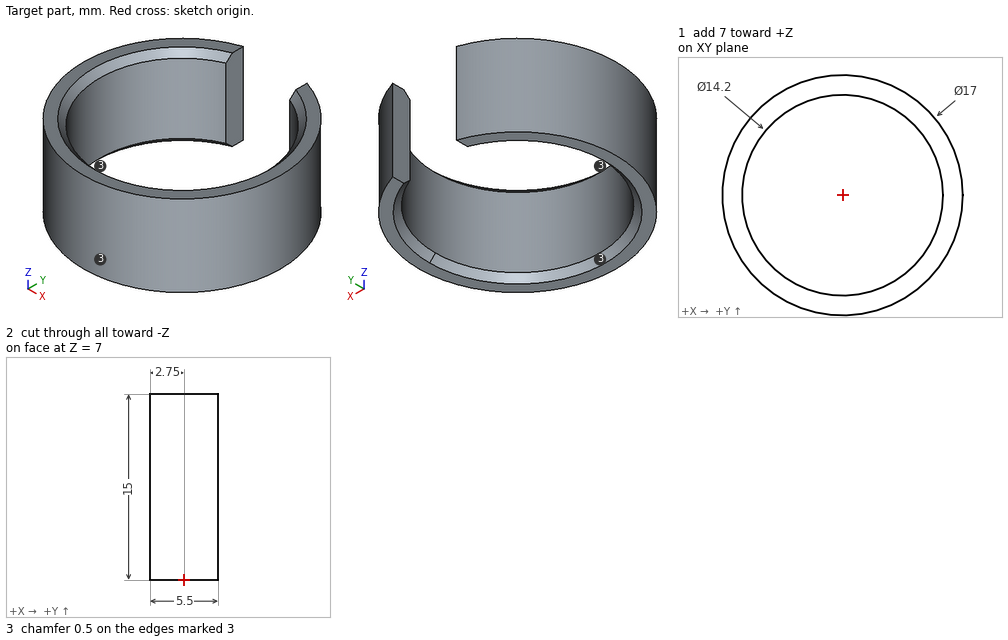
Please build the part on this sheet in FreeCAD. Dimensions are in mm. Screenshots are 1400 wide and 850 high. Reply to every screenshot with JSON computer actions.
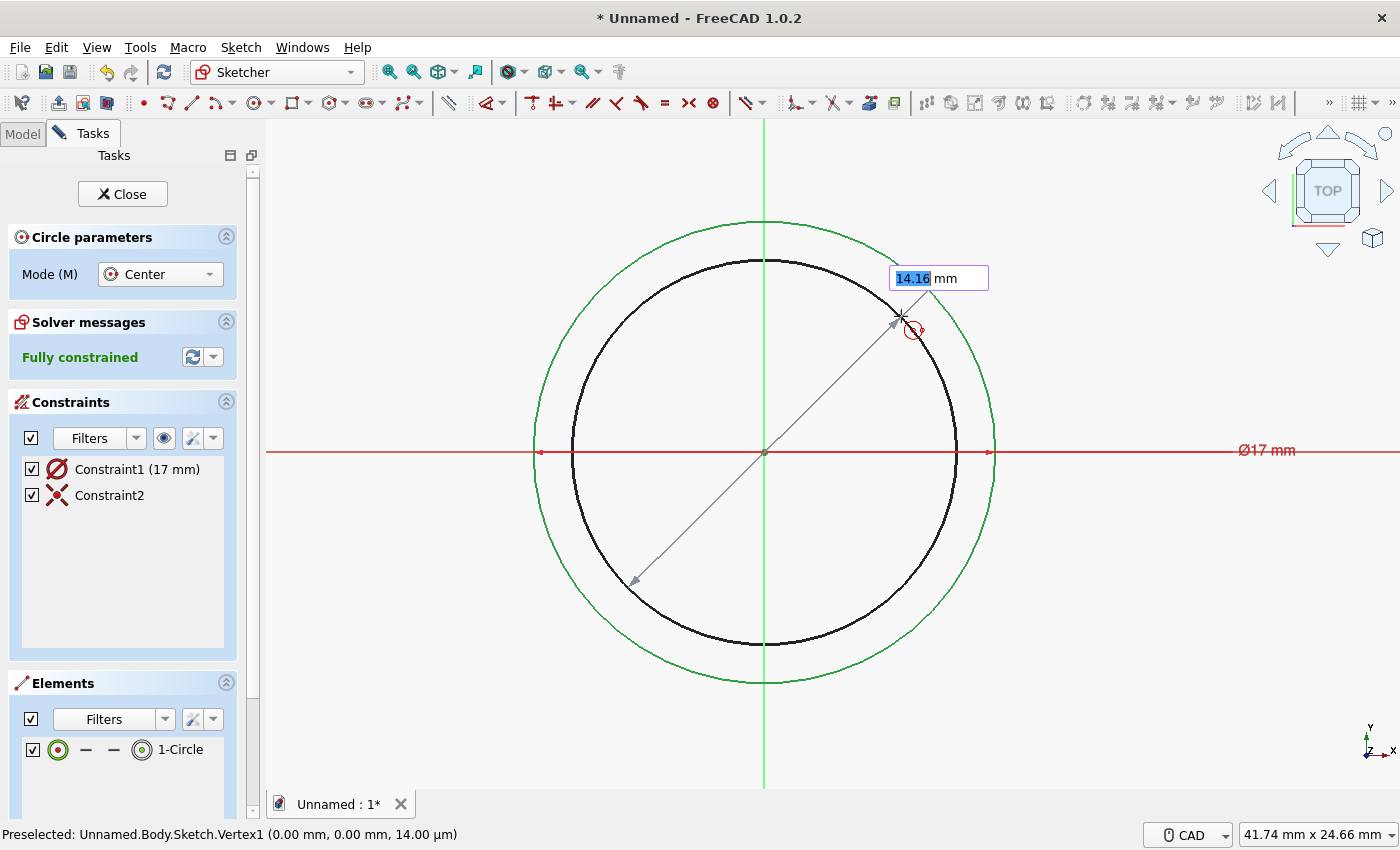
{"action": "type", "text": "14.2"}
{"action": "key", "text": "Return"}
{"action": "key", "text": "Escape"}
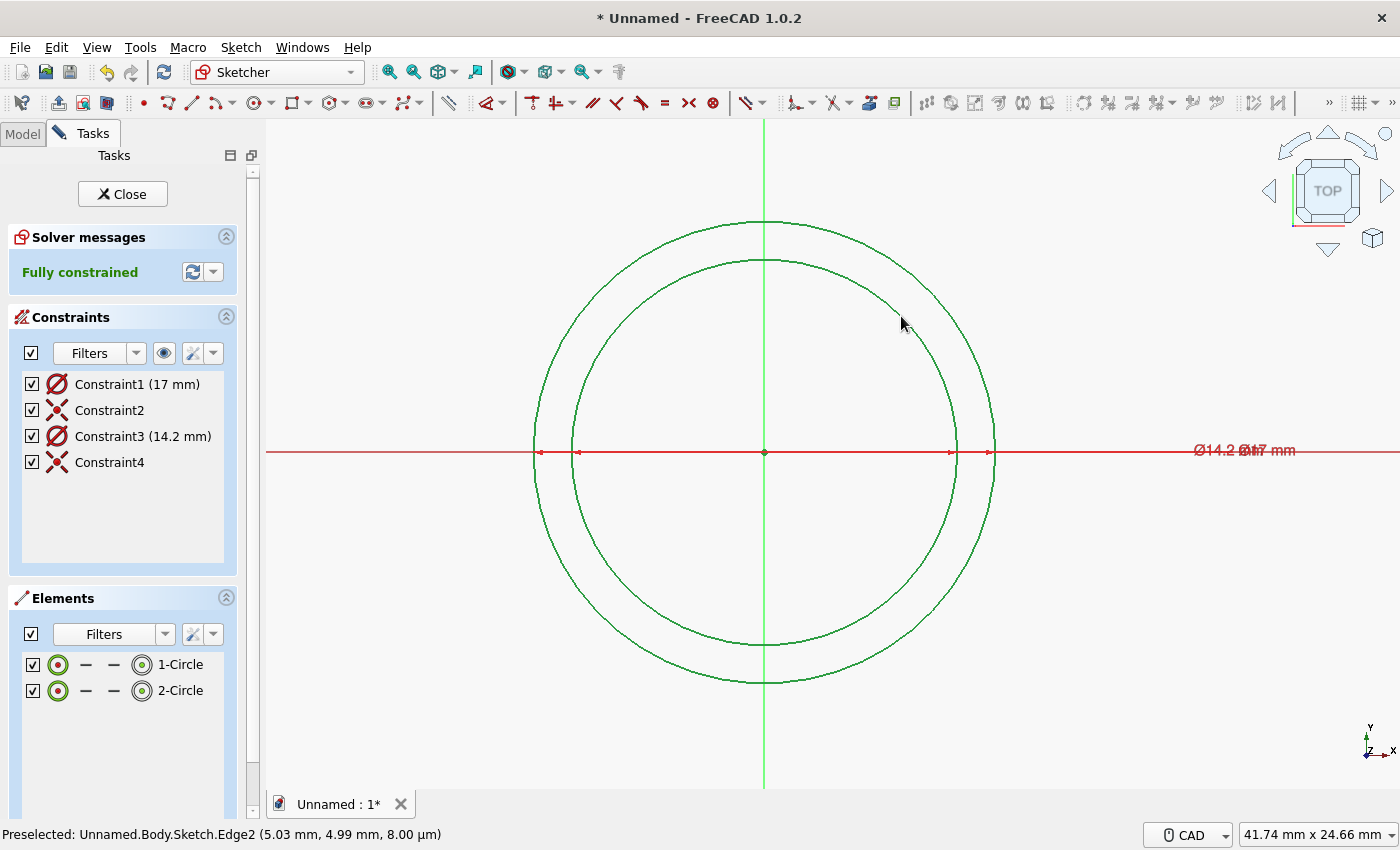
{"action": "left_click", "coordinate": [123, 194]}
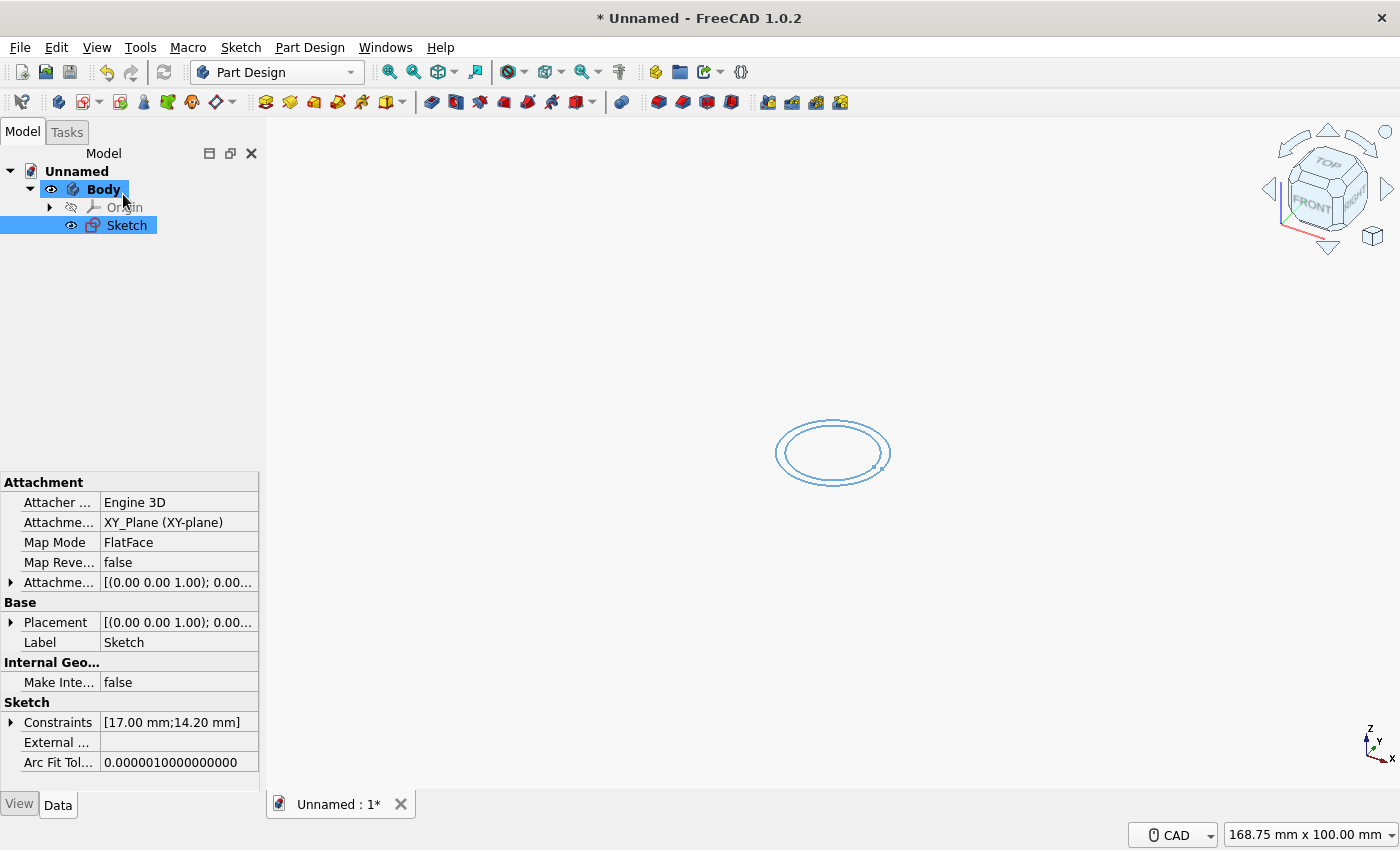
{"action": "left_click", "coordinate": [266, 102]}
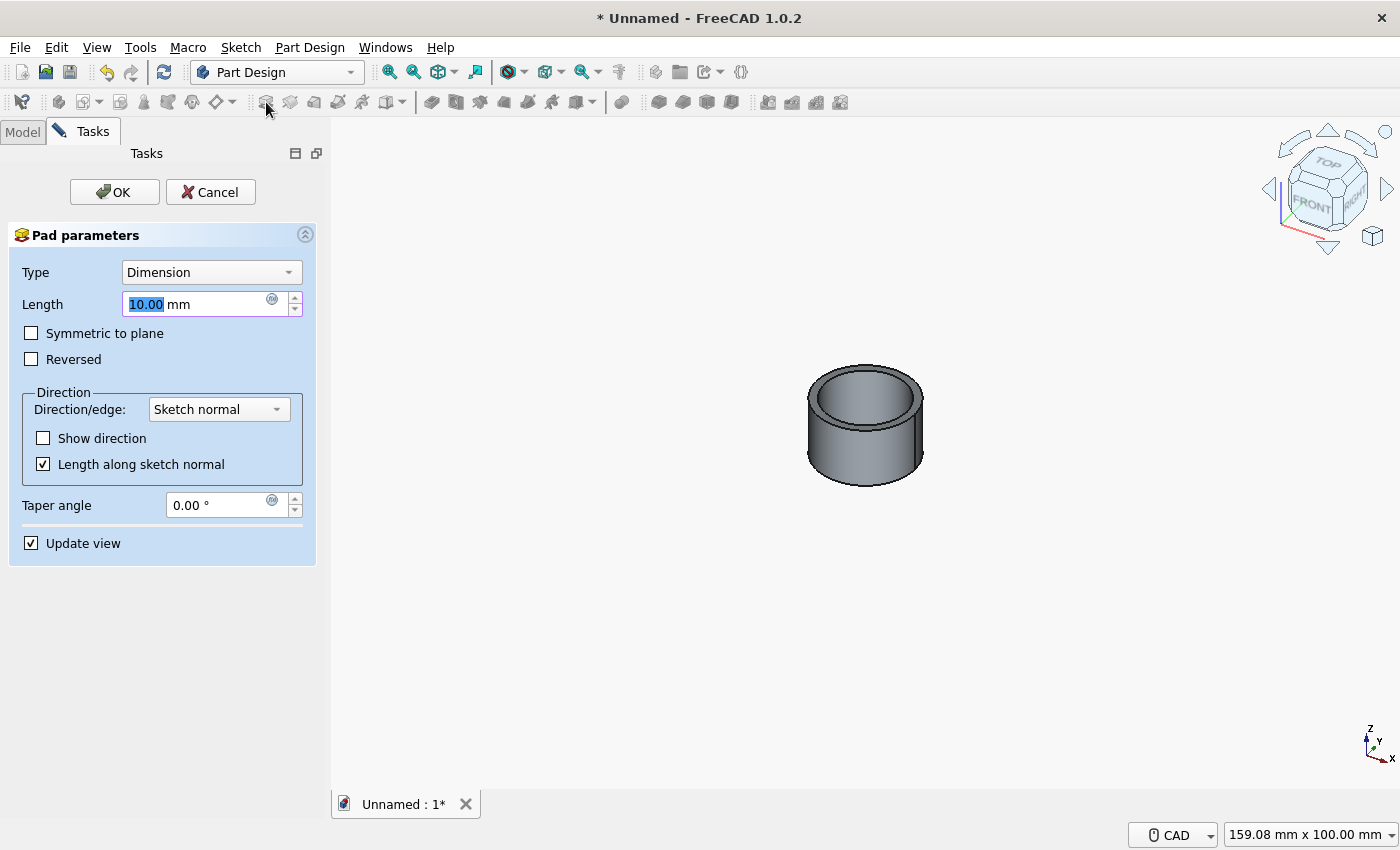
{"action": "type", "text": "7"}
{"action": "key", "text": "Tab"}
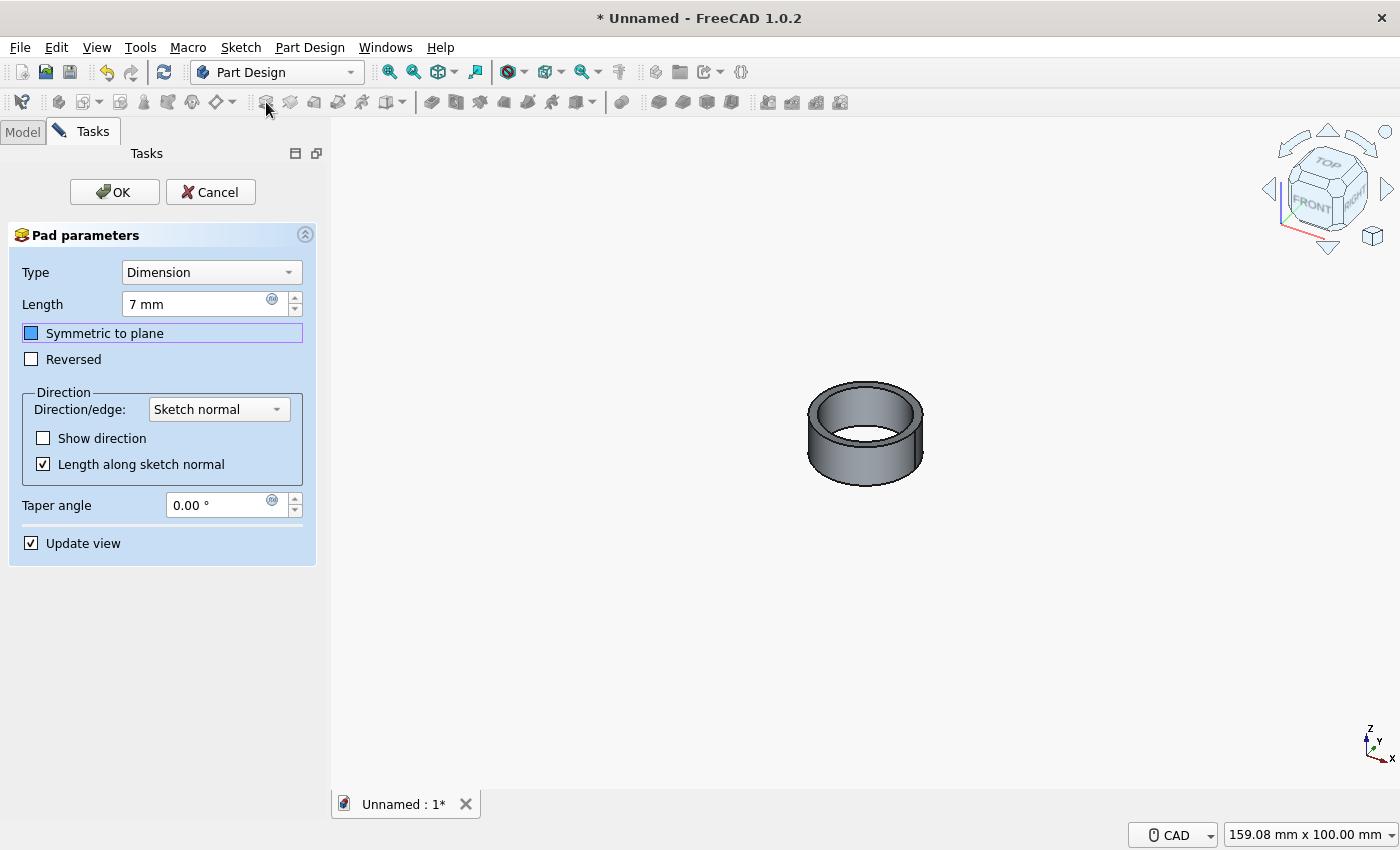
{"action": "left_click", "coordinate": [115, 192]}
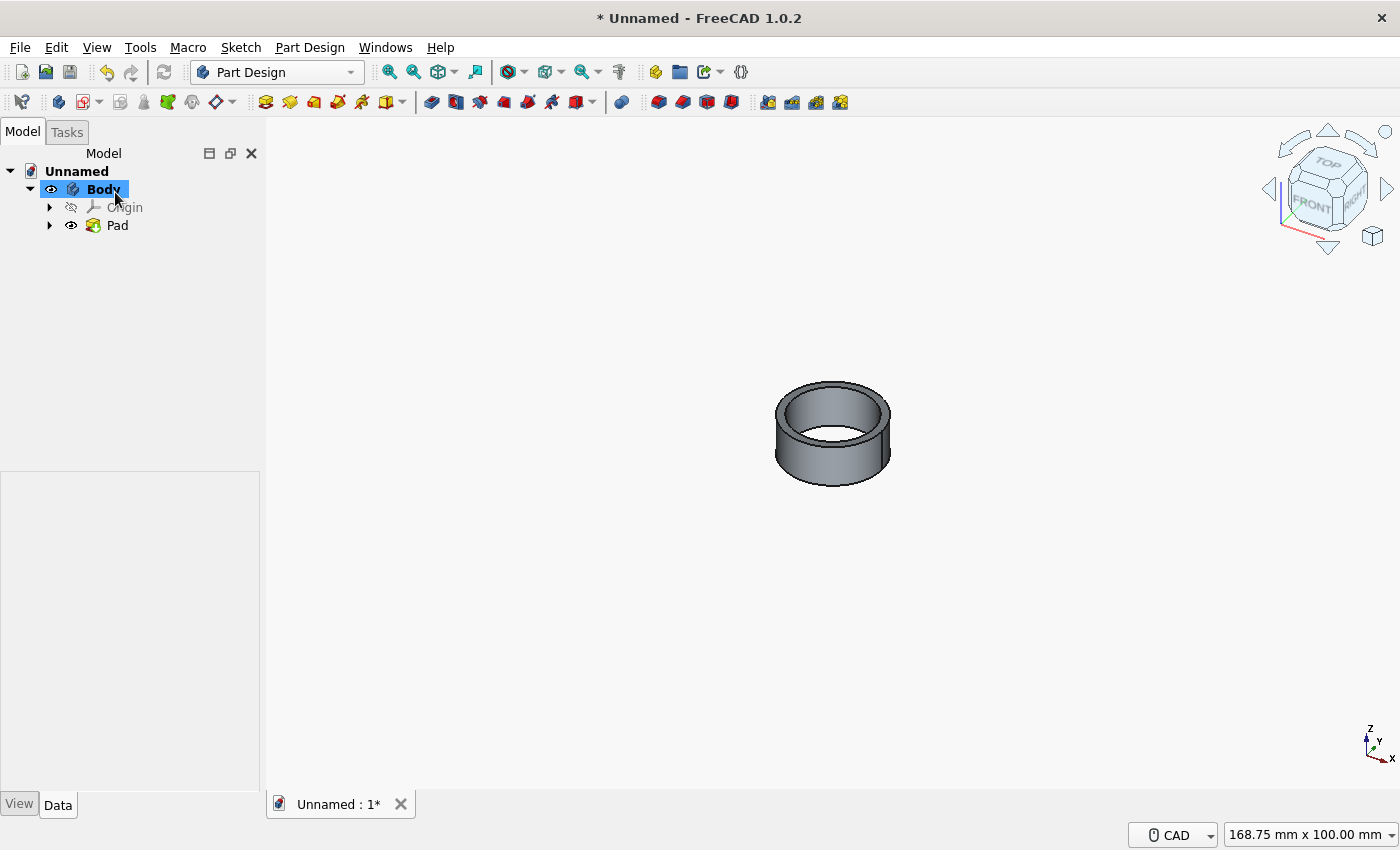
{"action": "left_click", "coordinate": [390, 72]}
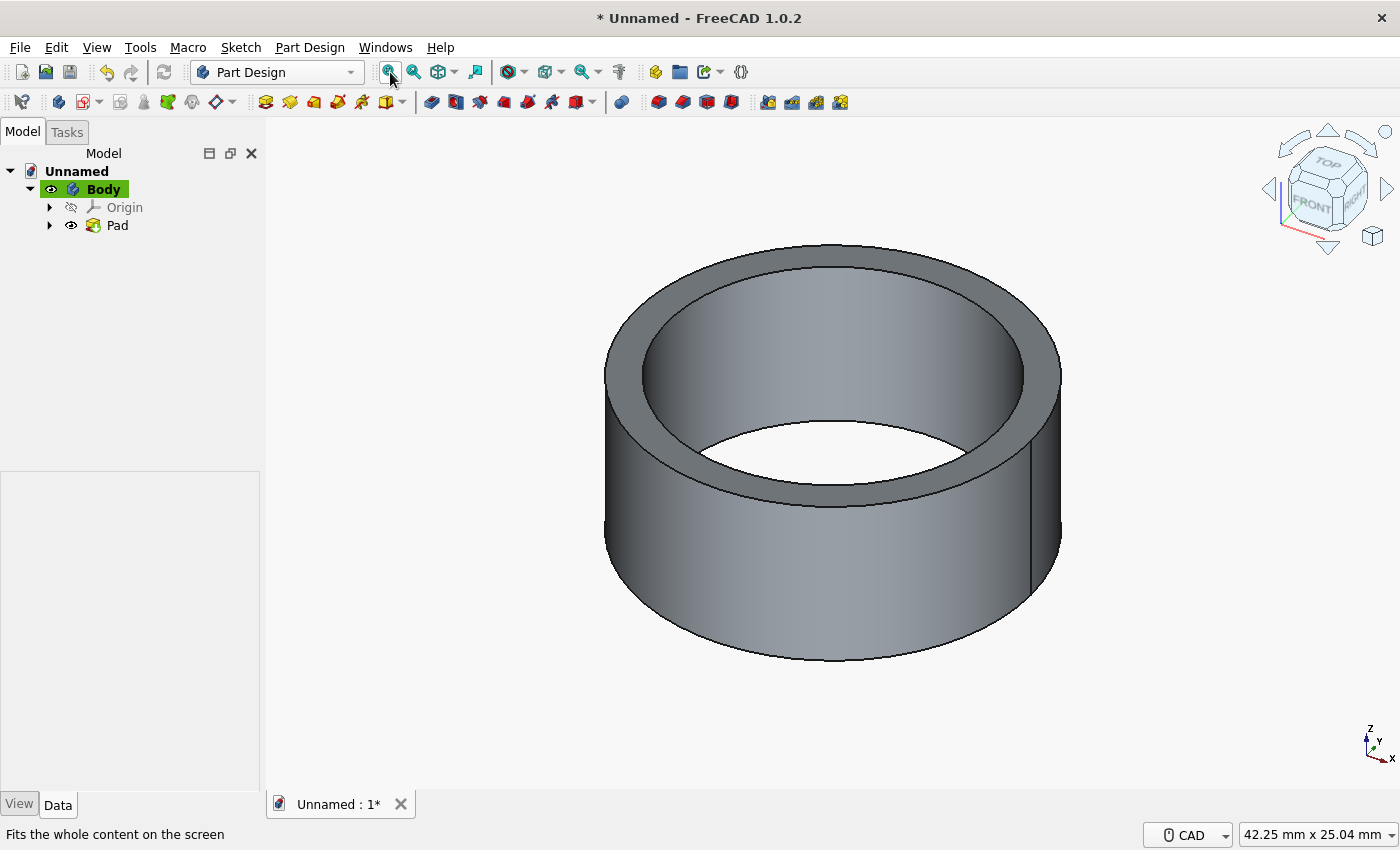
{"action": "left_click", "coordinate": [874, 259]}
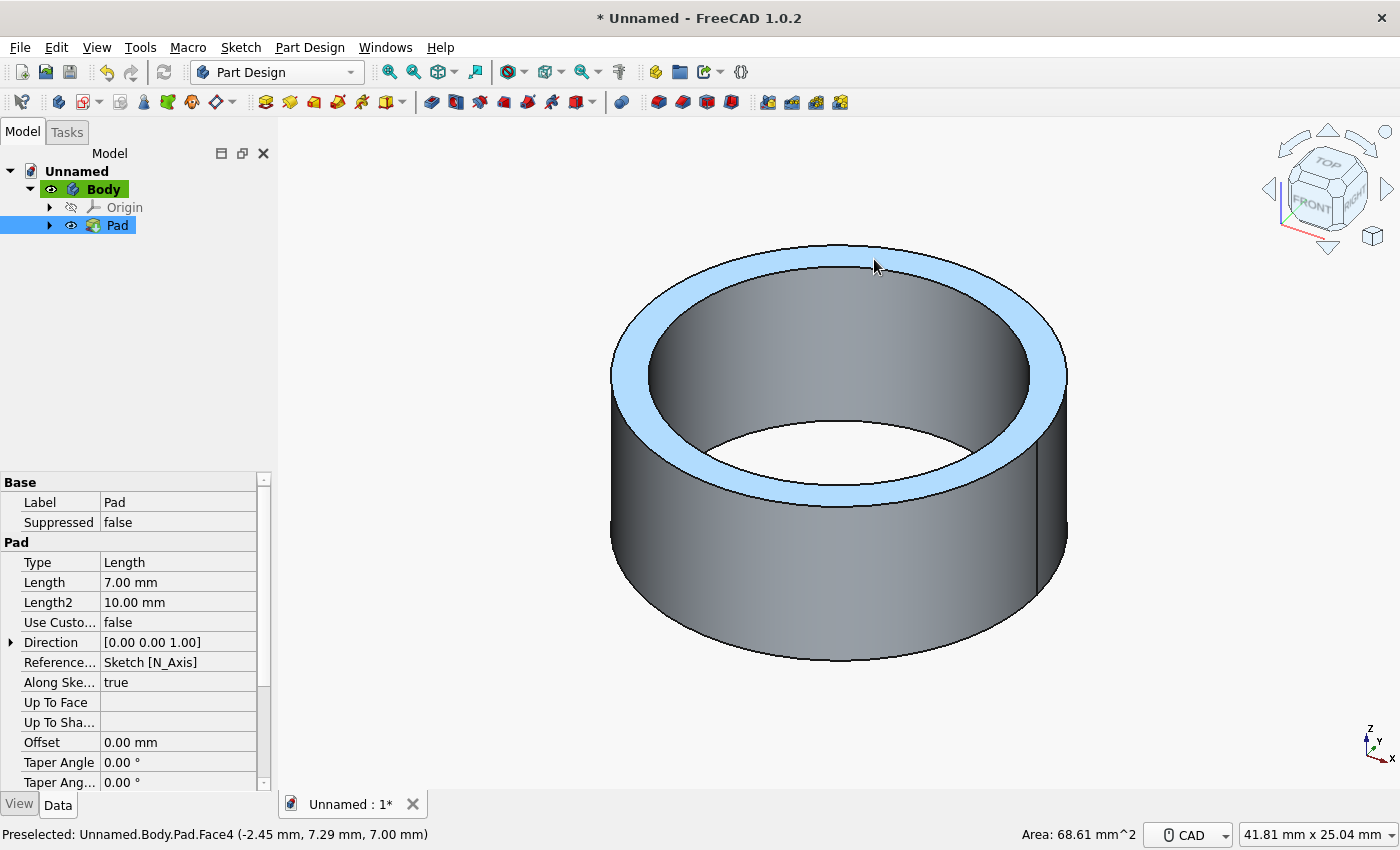
{"action": "left_click", "coordinate": [84, 102]}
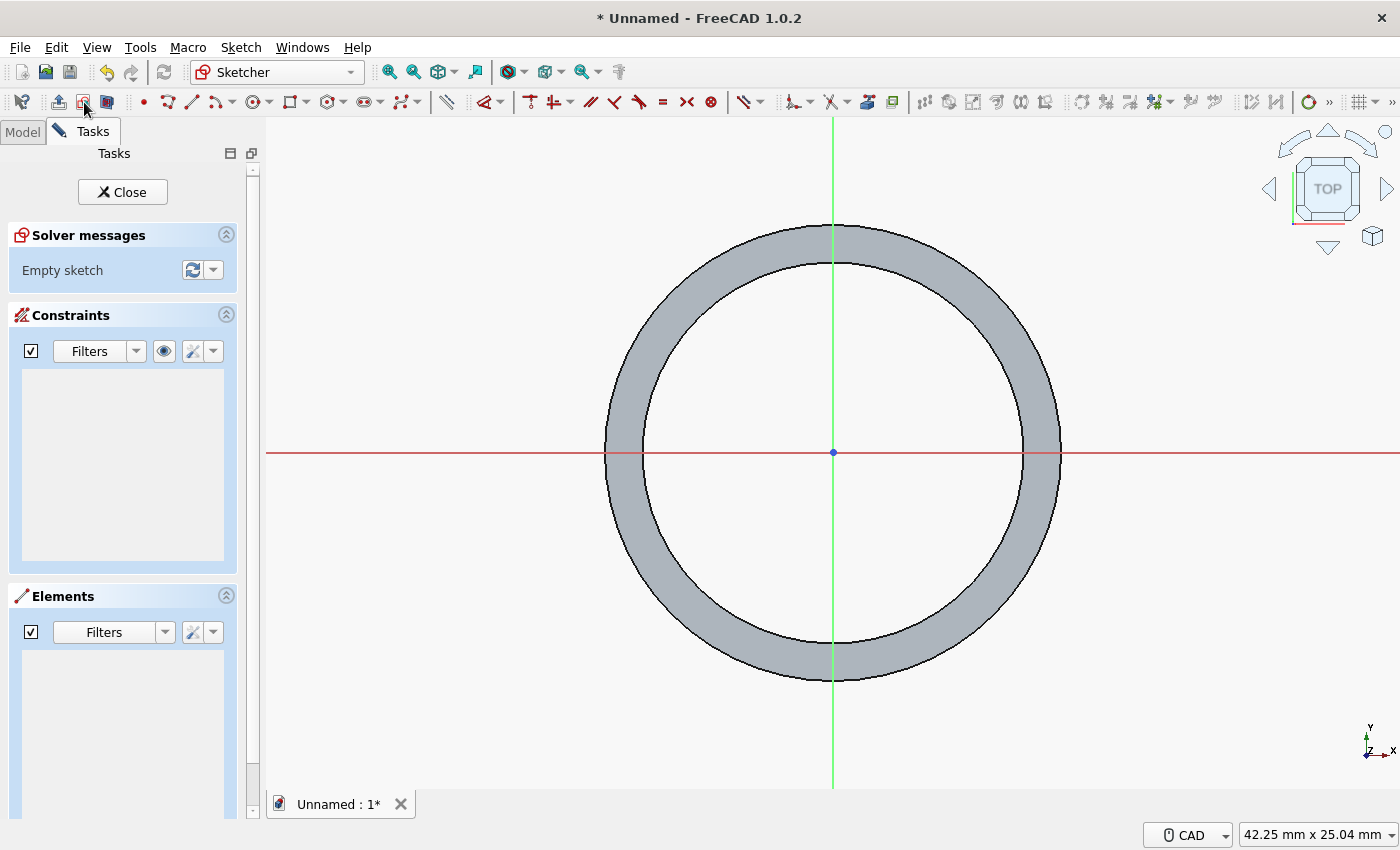
{"action": "scroll", "coordinate": [455, 761], "scroll_direction": "down", "scroll_amount": 1}